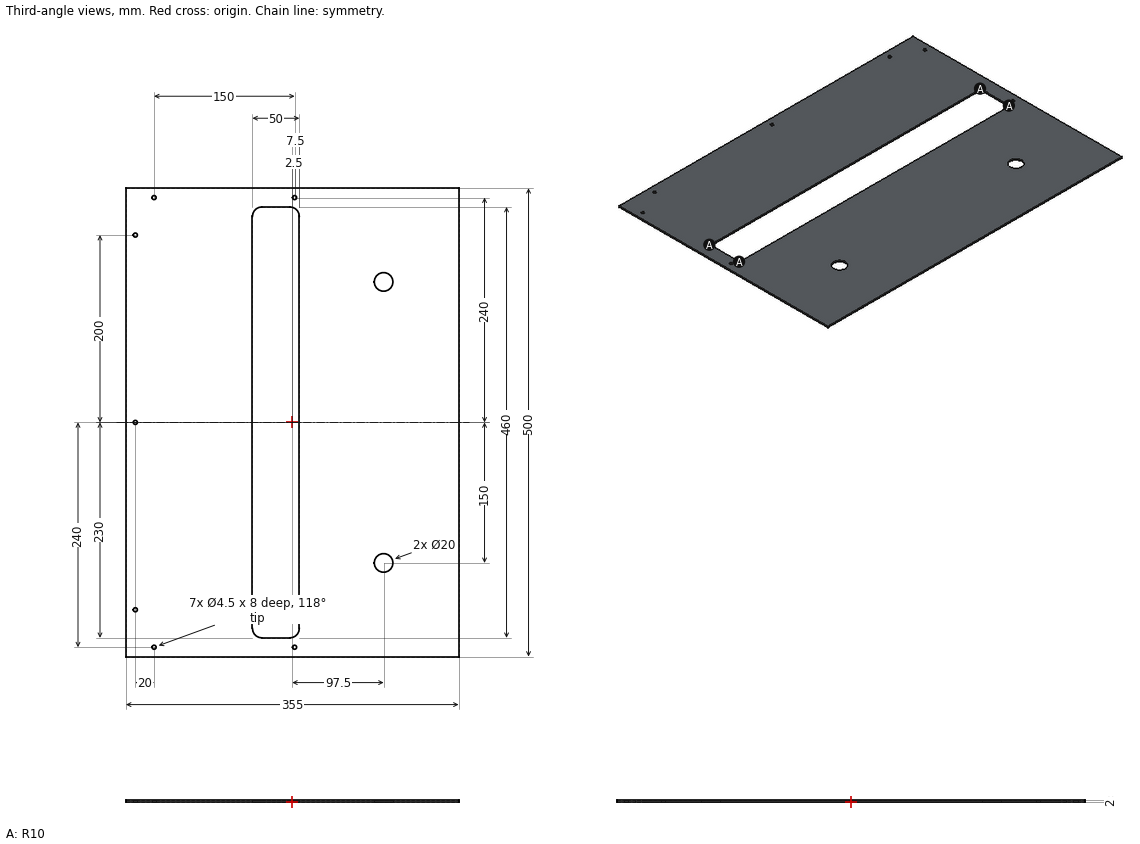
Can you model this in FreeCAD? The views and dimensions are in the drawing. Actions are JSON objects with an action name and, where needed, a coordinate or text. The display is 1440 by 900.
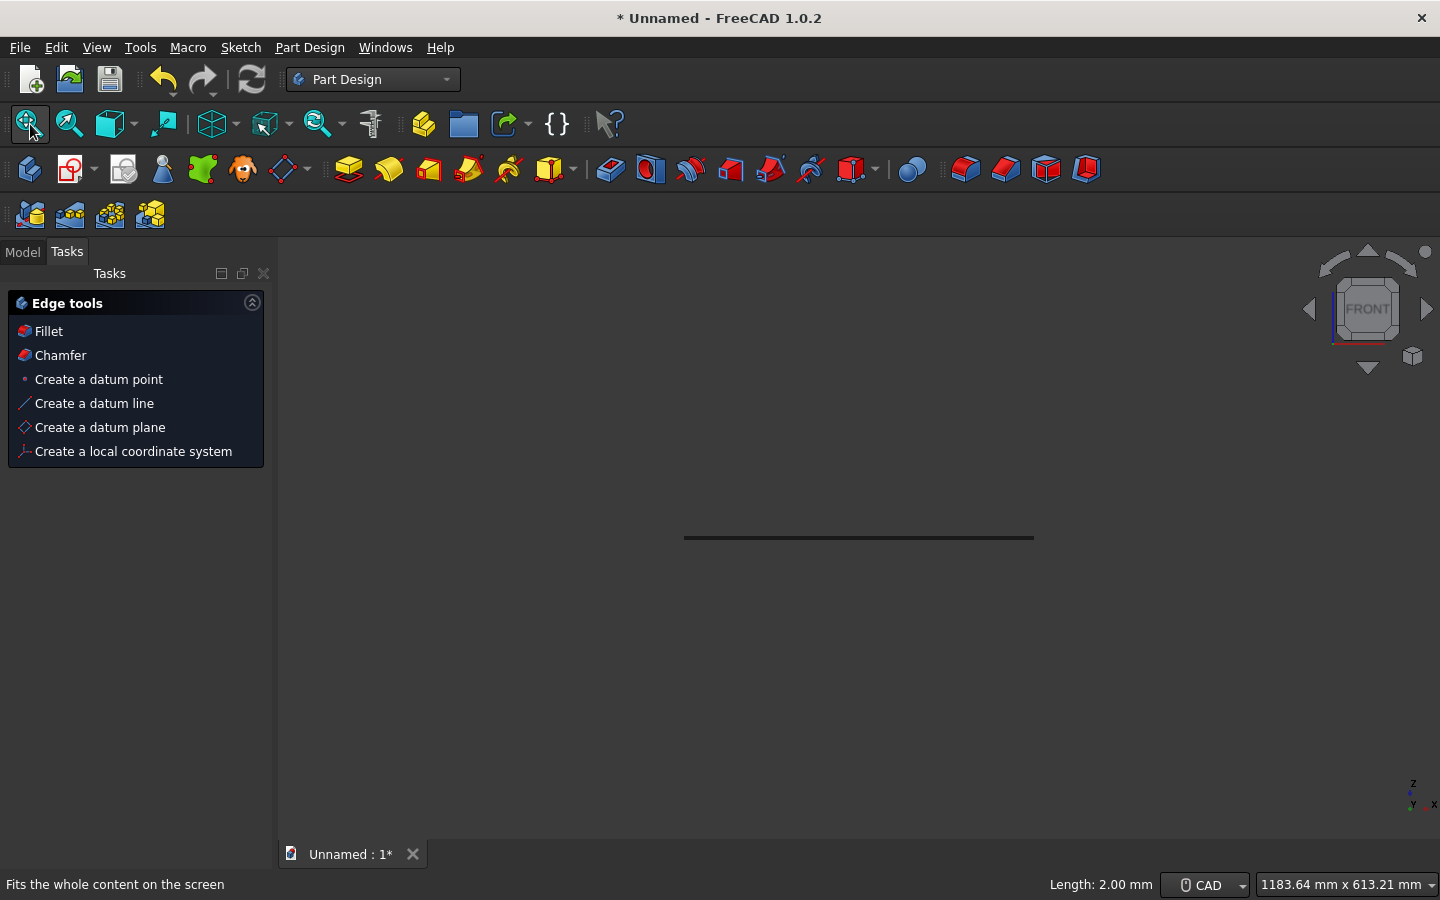
{"action": "scroll", "coordinate": [817, 537], "scroll_direction": "up", "scroll_amount": 15}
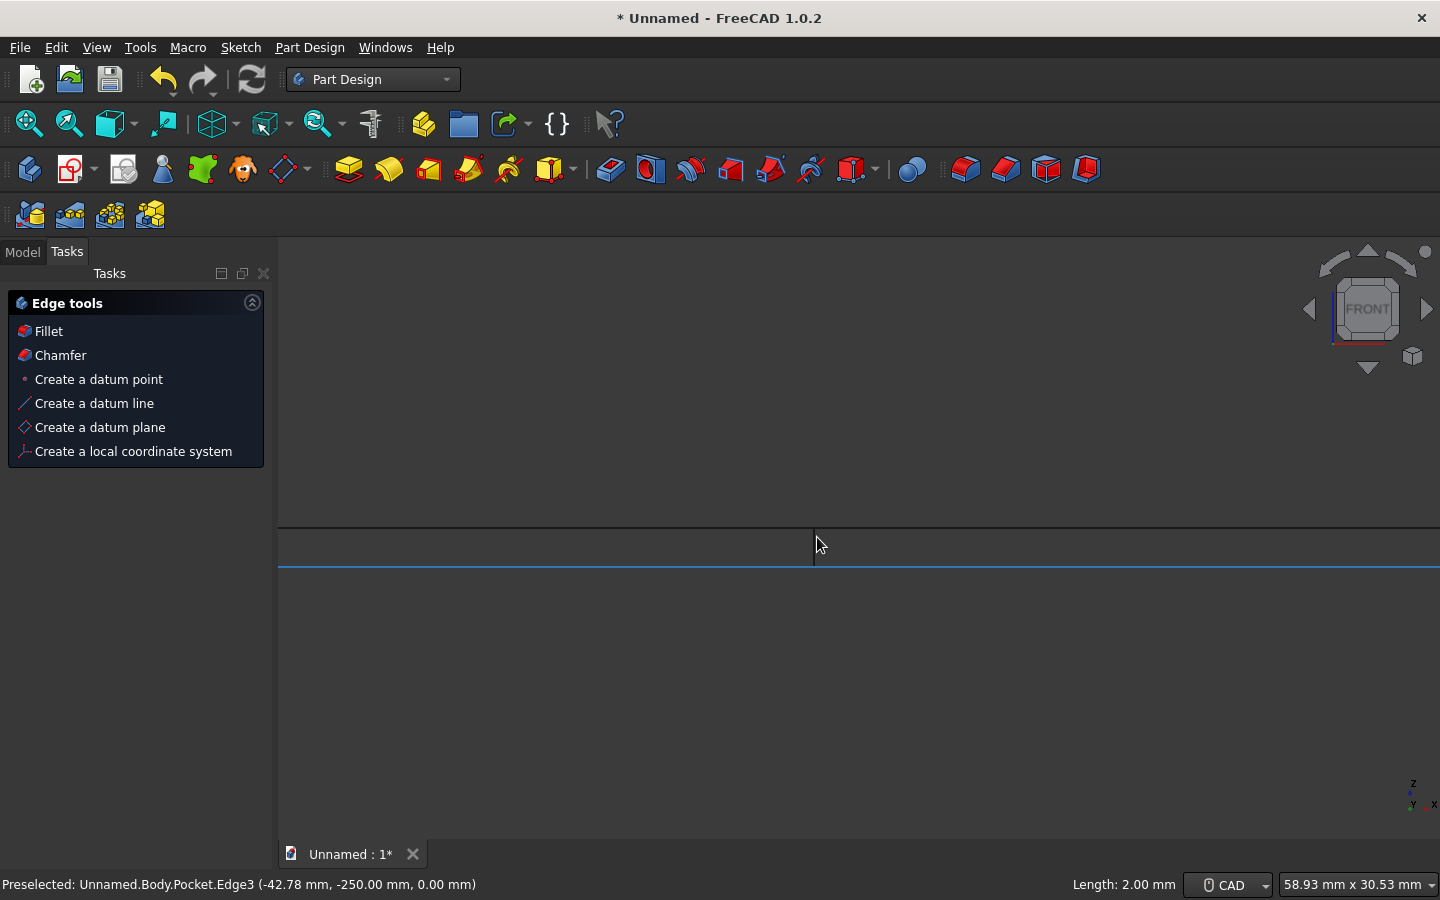
{"action": "left_click", "coordinate": [814, 547], "text": "ctrl"}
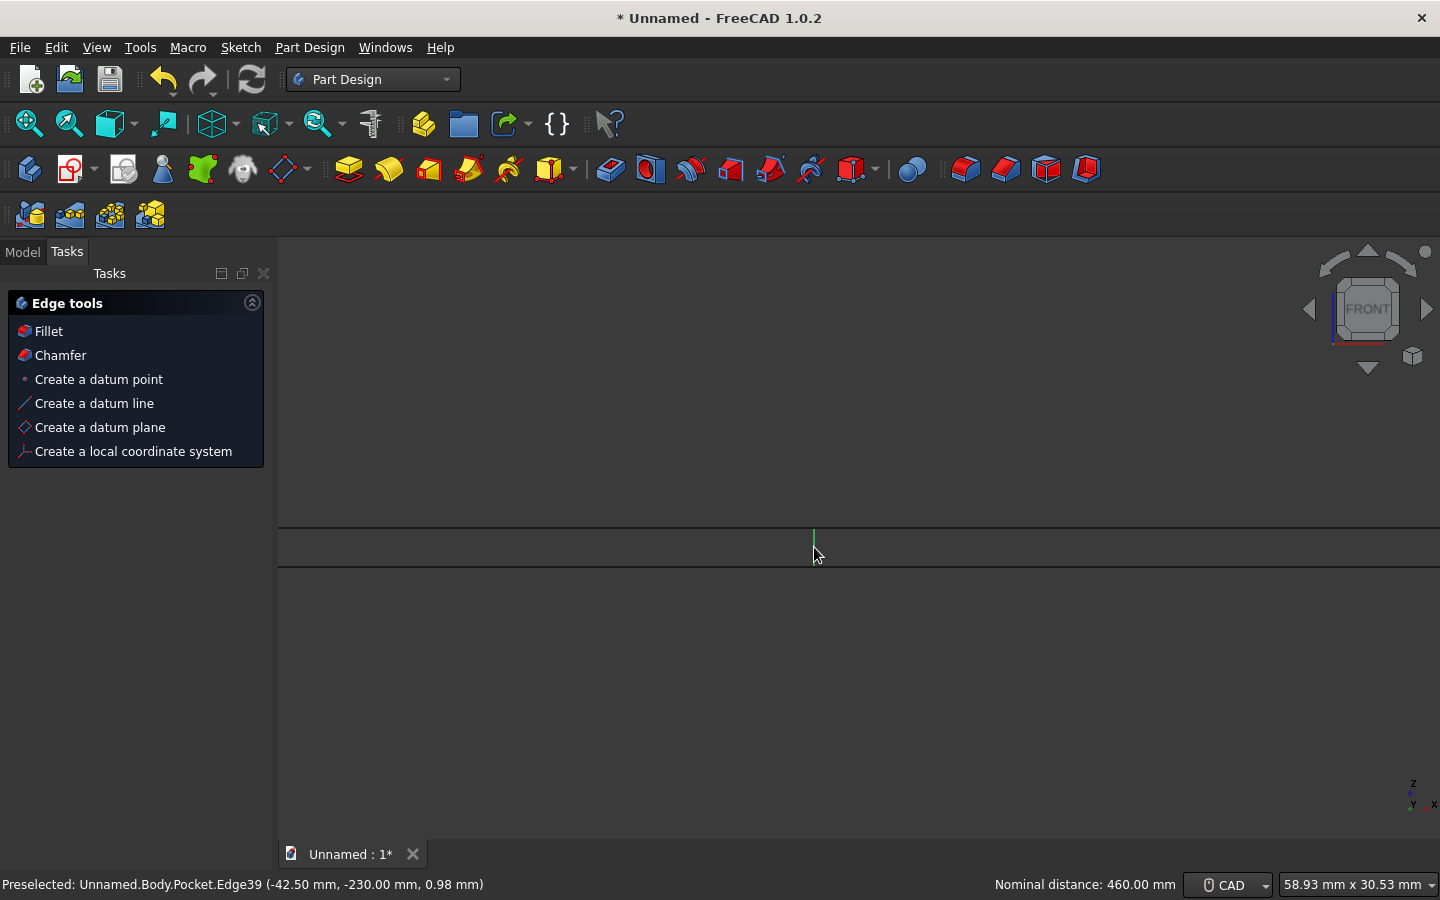
{"action": "left_click", "coordinate": [30, 124]}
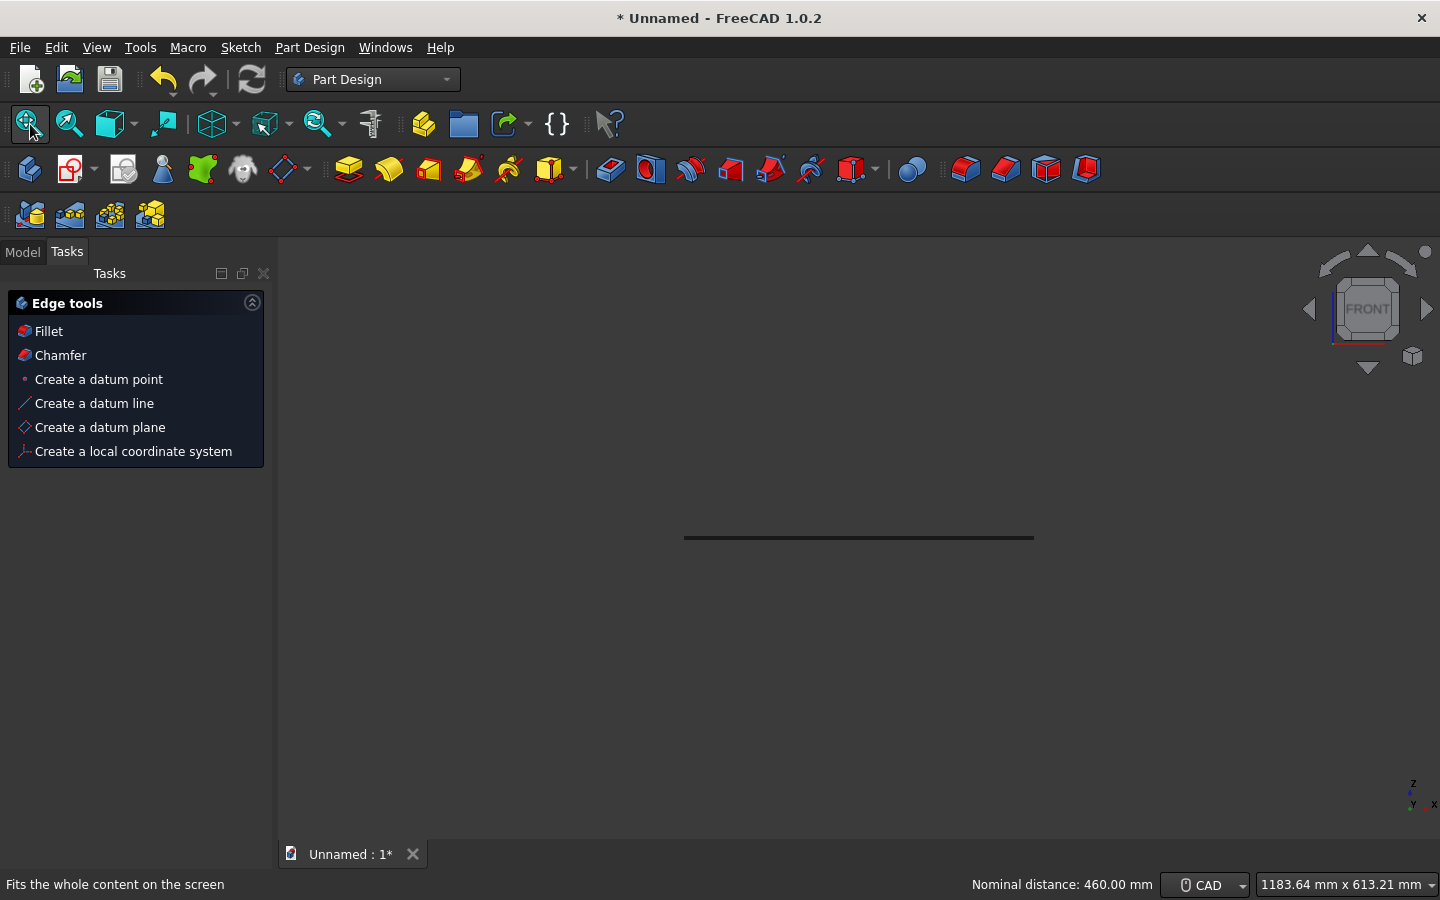
{"action": "key", "text": "3"}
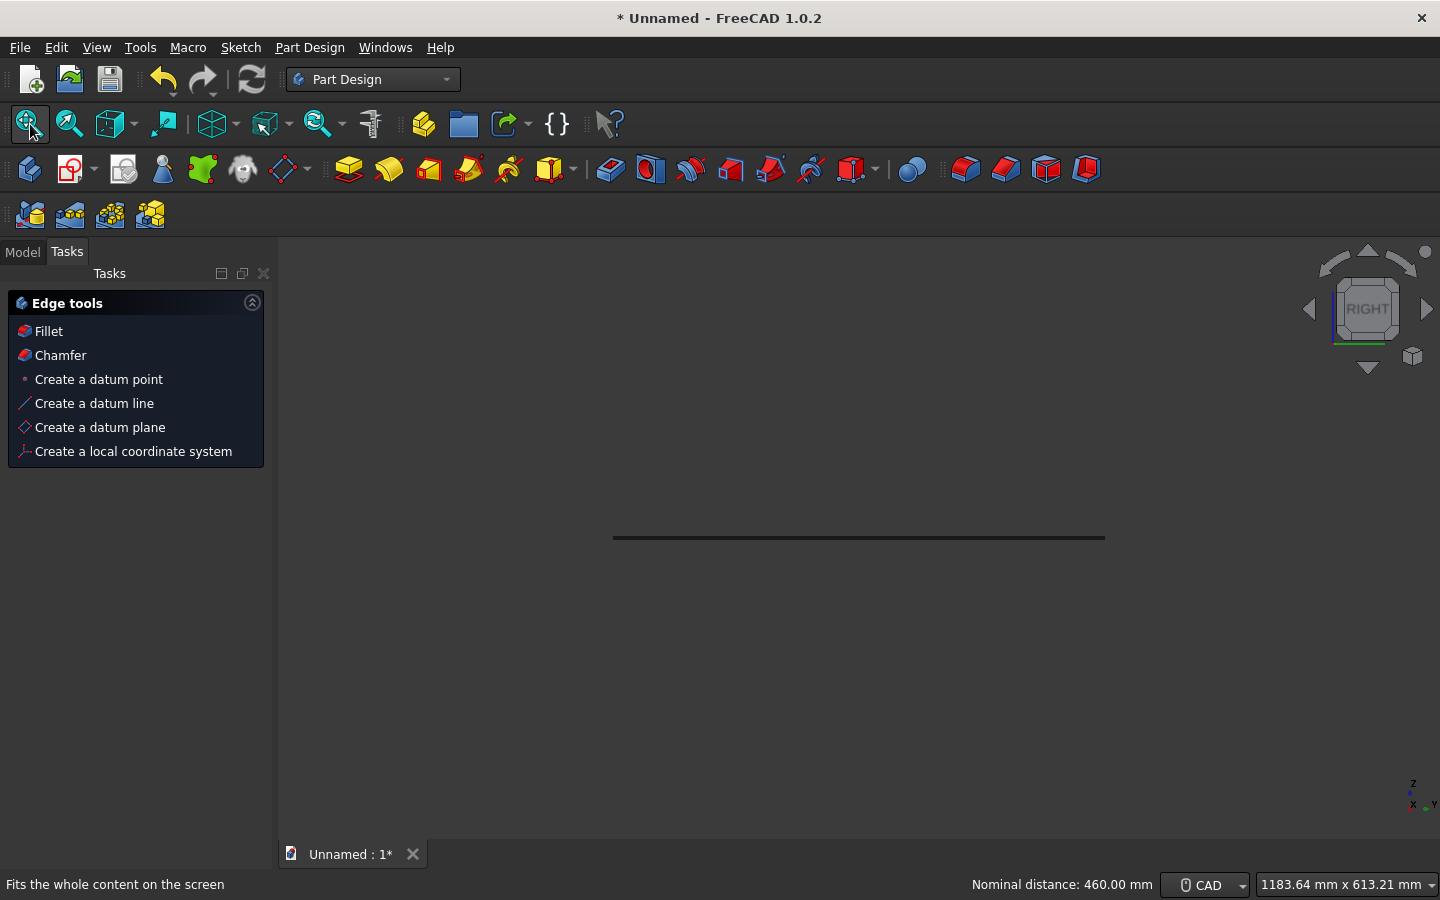
{"action": "key", "text": "v f"}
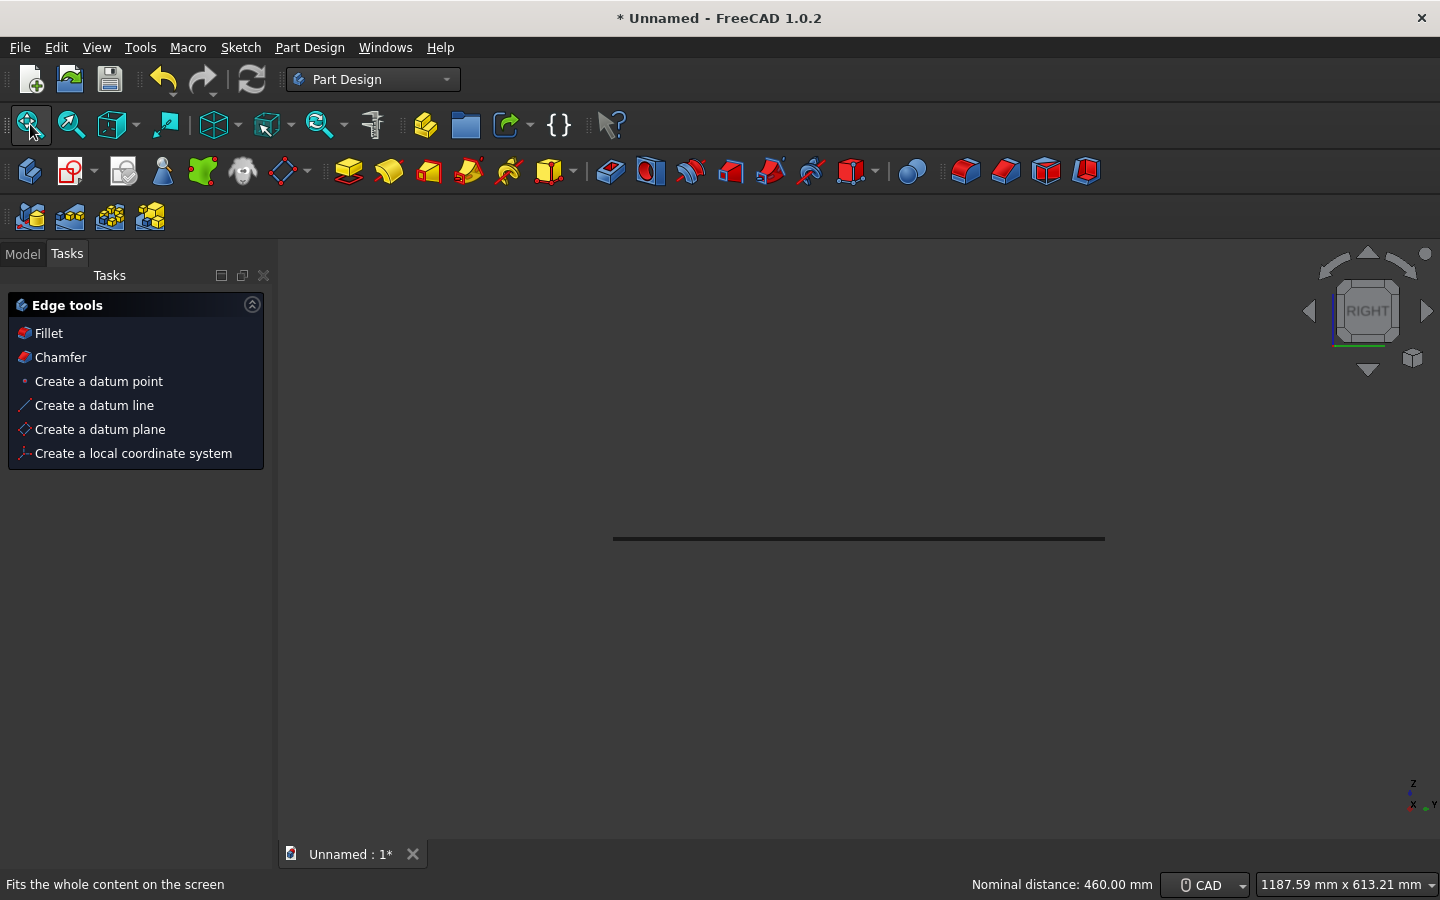
{"action": "scroll", "coordinate": [634, 538], "scroll_direction": "up", "scroll_amount": 15}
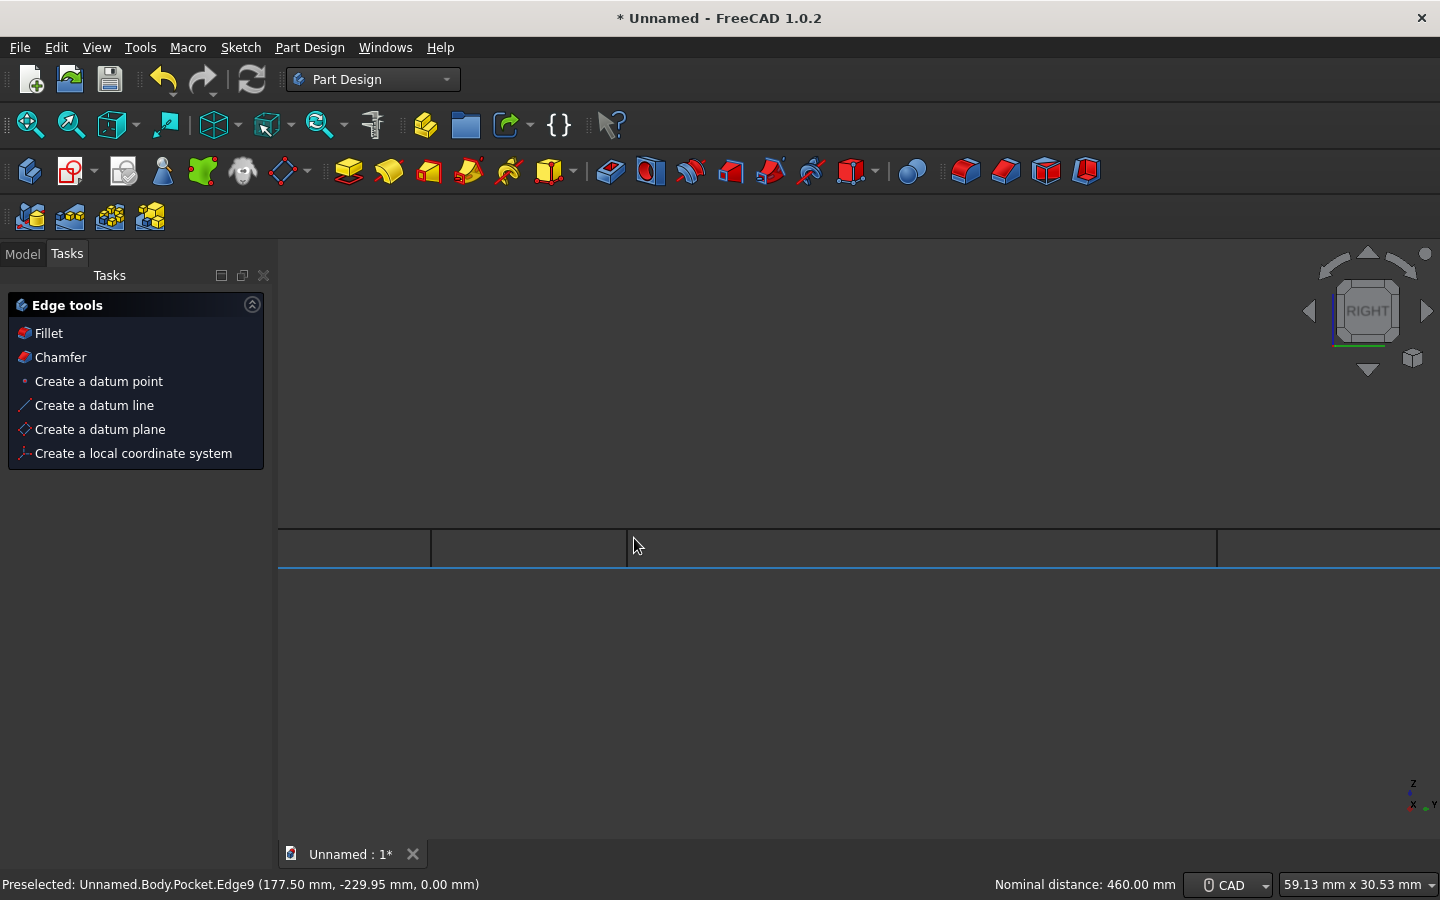
{"action": "left_click", "coordinate": [627, 548], "text": "ctrl"}